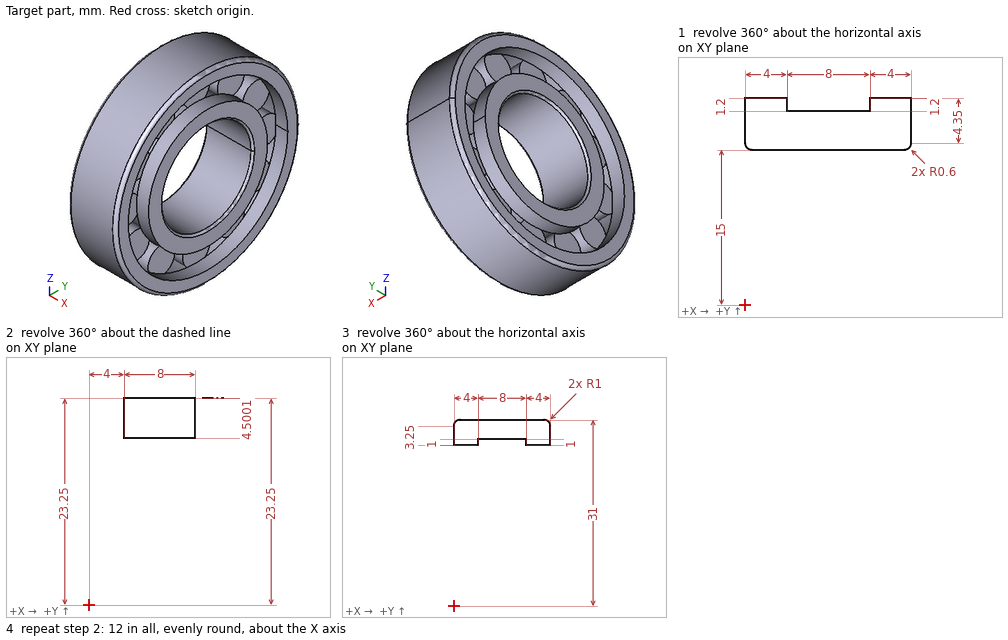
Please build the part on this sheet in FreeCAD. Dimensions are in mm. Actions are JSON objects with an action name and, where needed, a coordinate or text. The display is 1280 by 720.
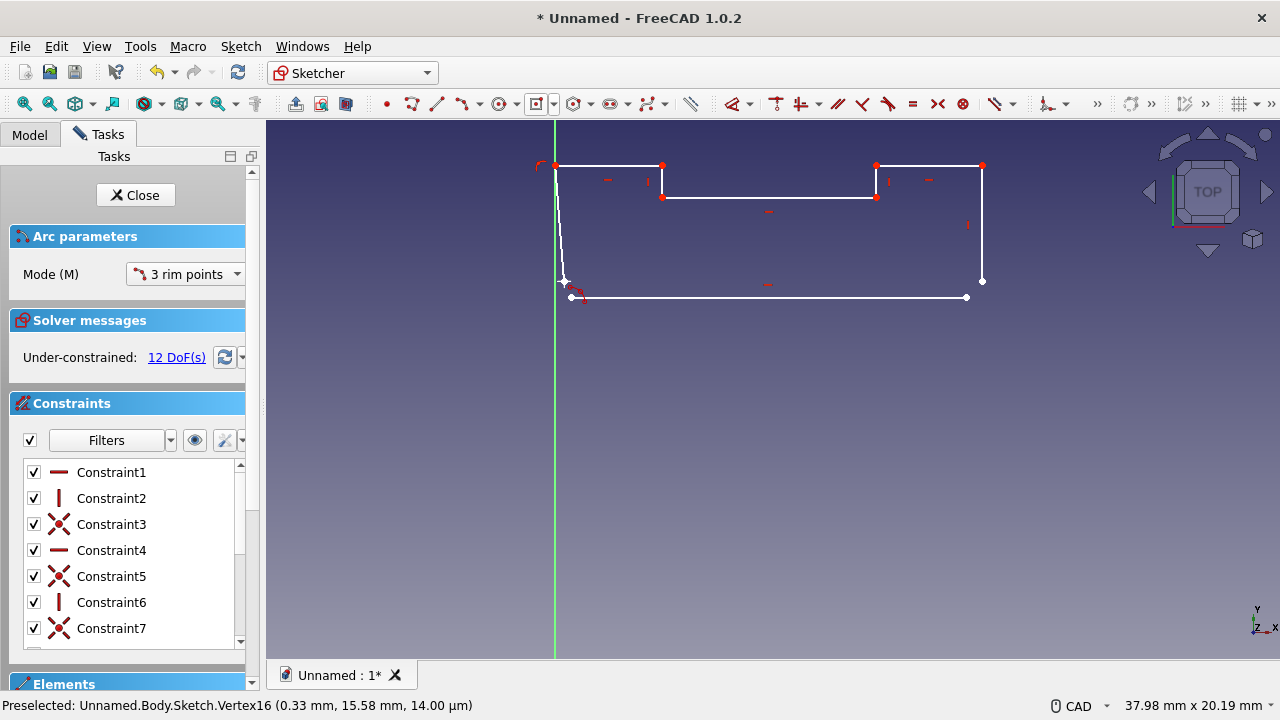
{"action": "left_click", "coordinate": [966, 298]}
{"action": "left_click", "coordinate": [982, 282]}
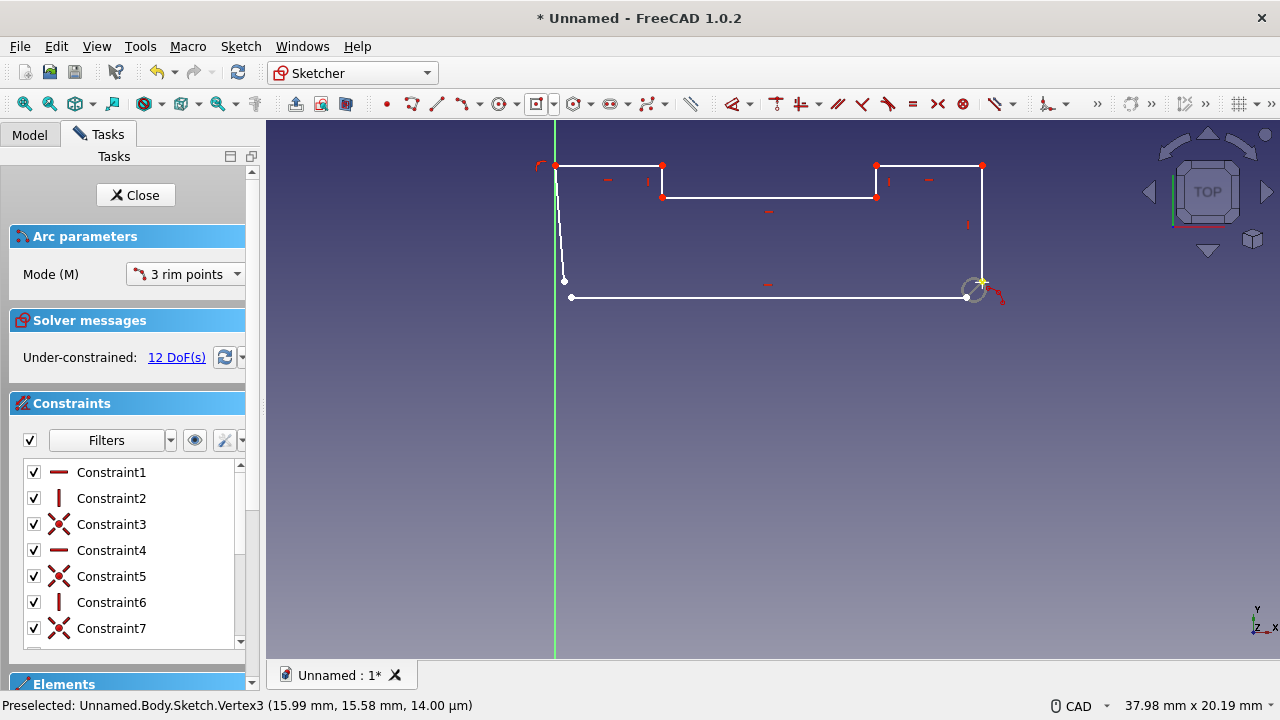
{"action": "scroll", "coordinate": [978, 293], "scroll_direction": "up", "scroll_amount": 7}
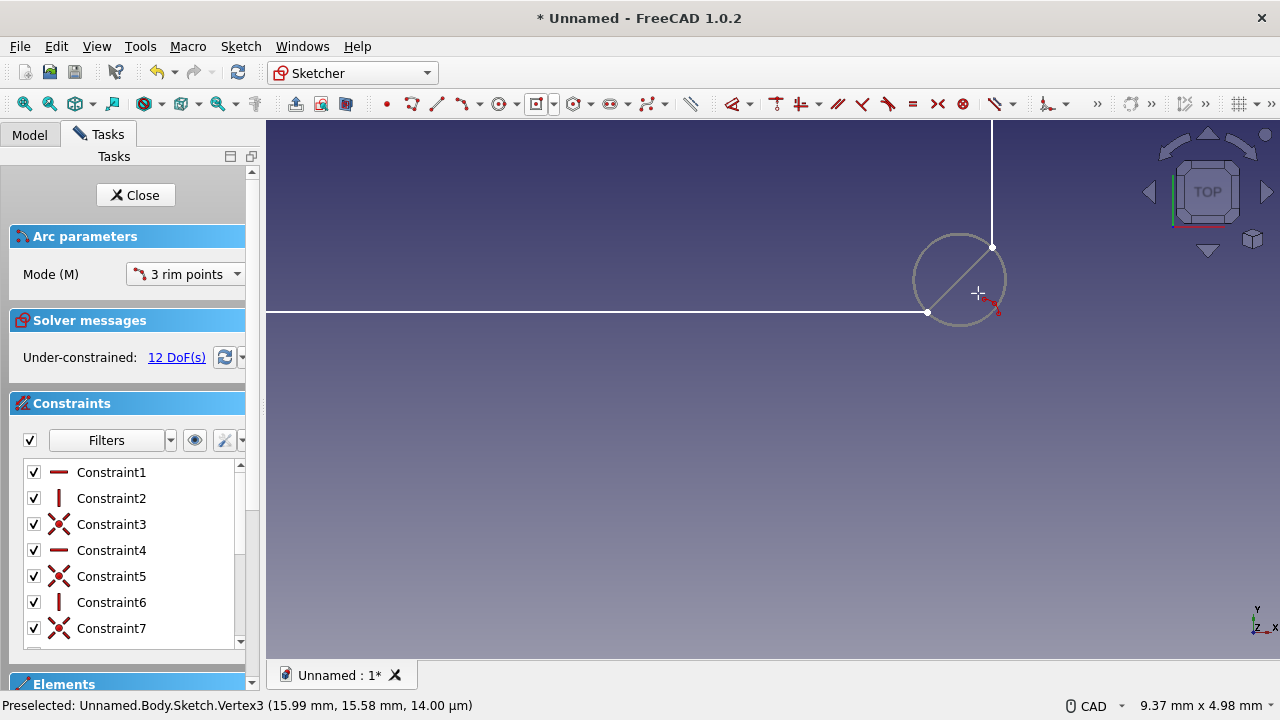
{"action": "left_click", "coordinate": [974, 291]}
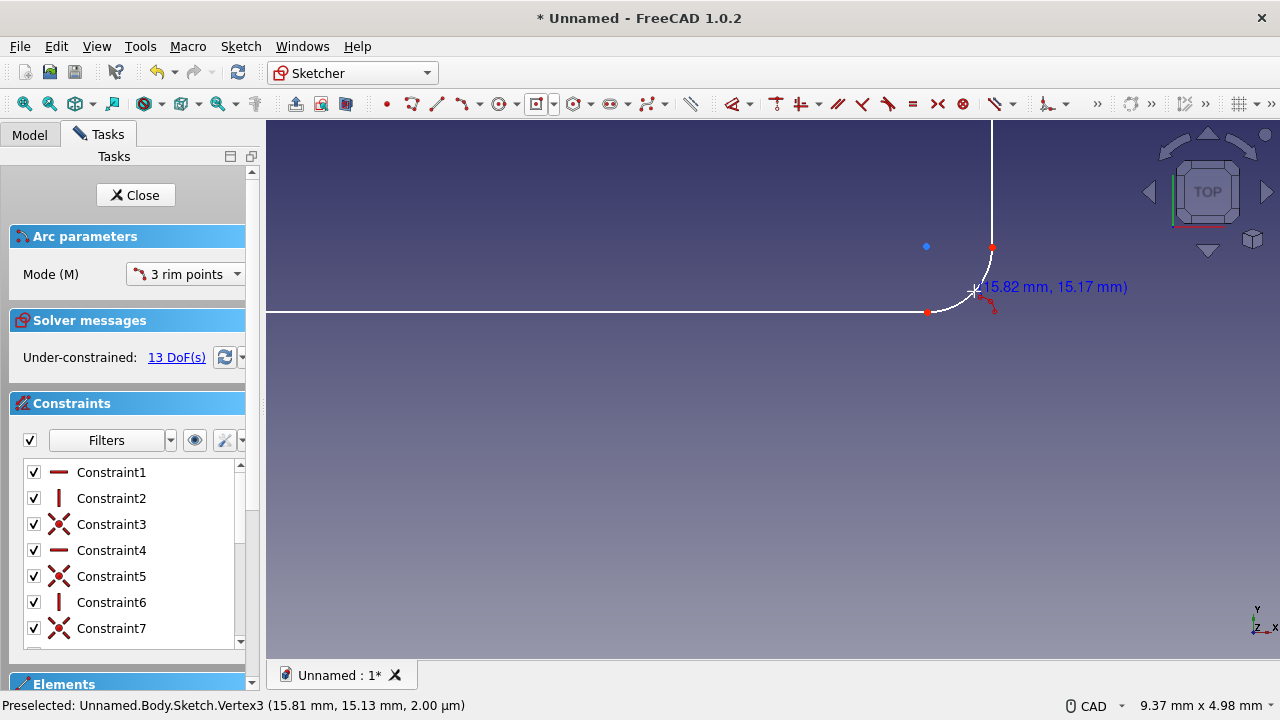
{"action": "scroll", "coordinate": [819, 298], "scroll_direction": "down", "scroll_amount": 9}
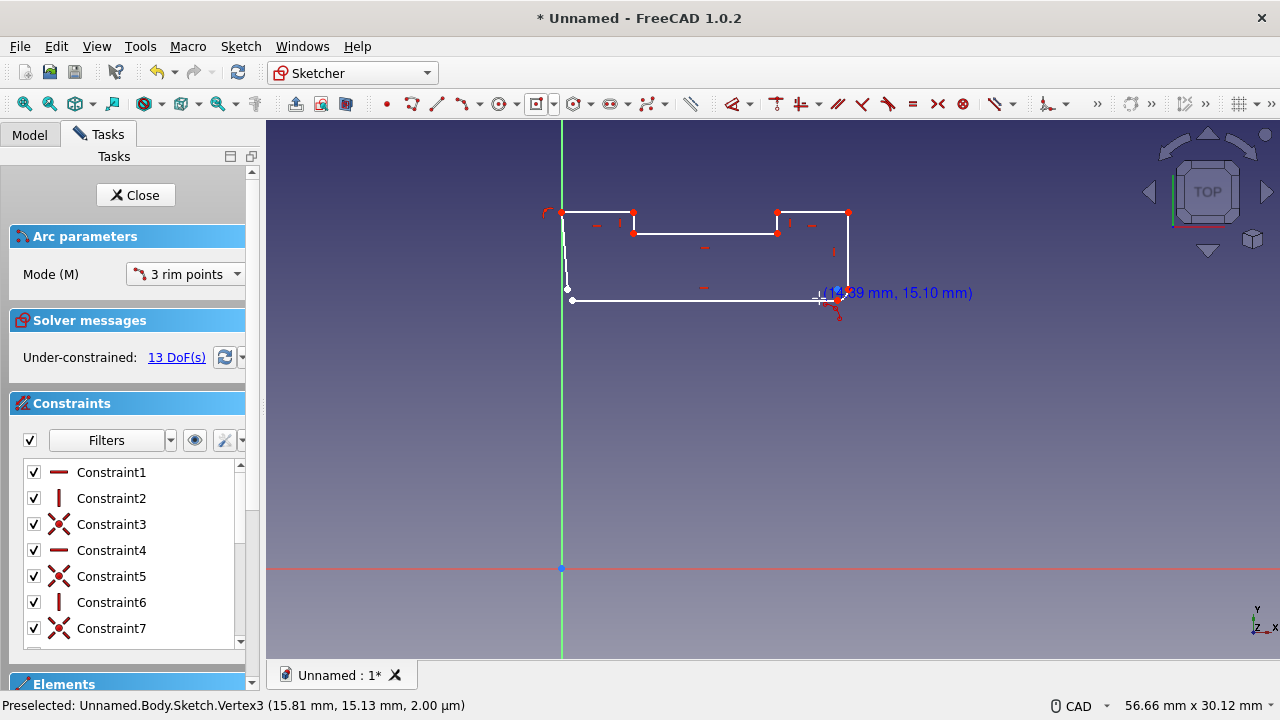
{"action": "left_click", "coordinate": [568, 290]}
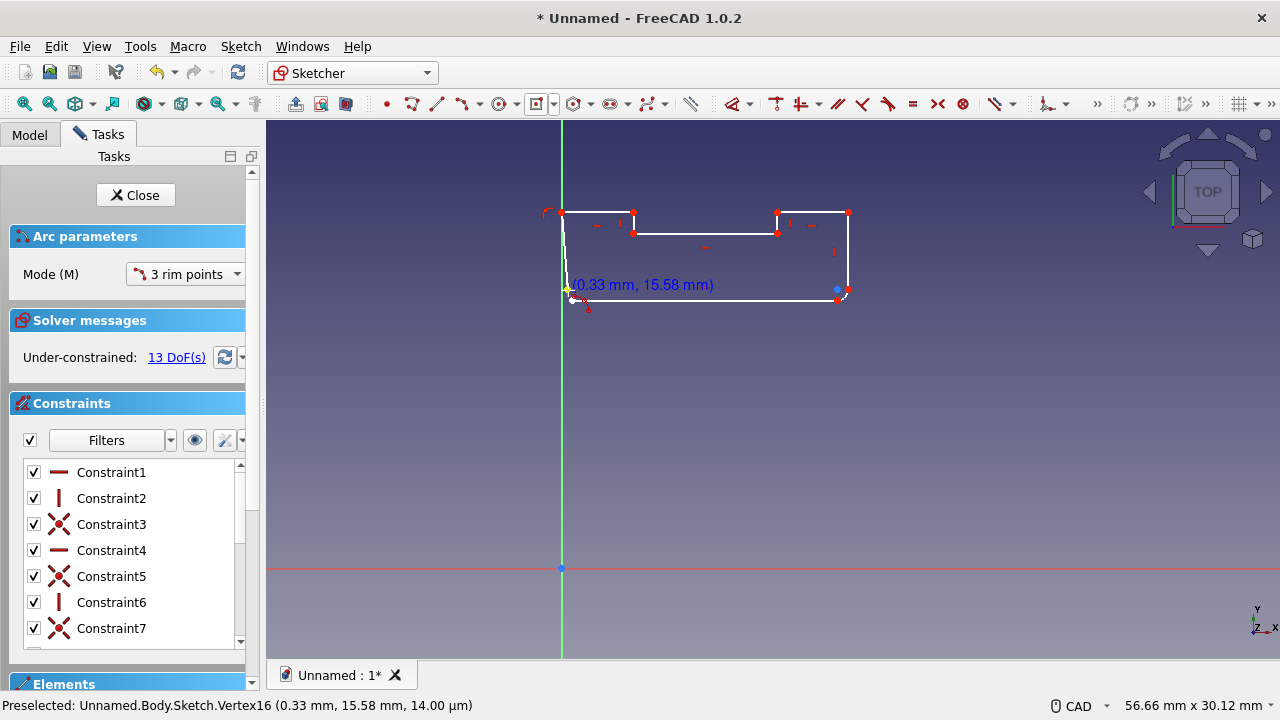
{"action": "scroll", "coordinate": [573, 300], "scroll_direction": "up", "scroll_amount": 2}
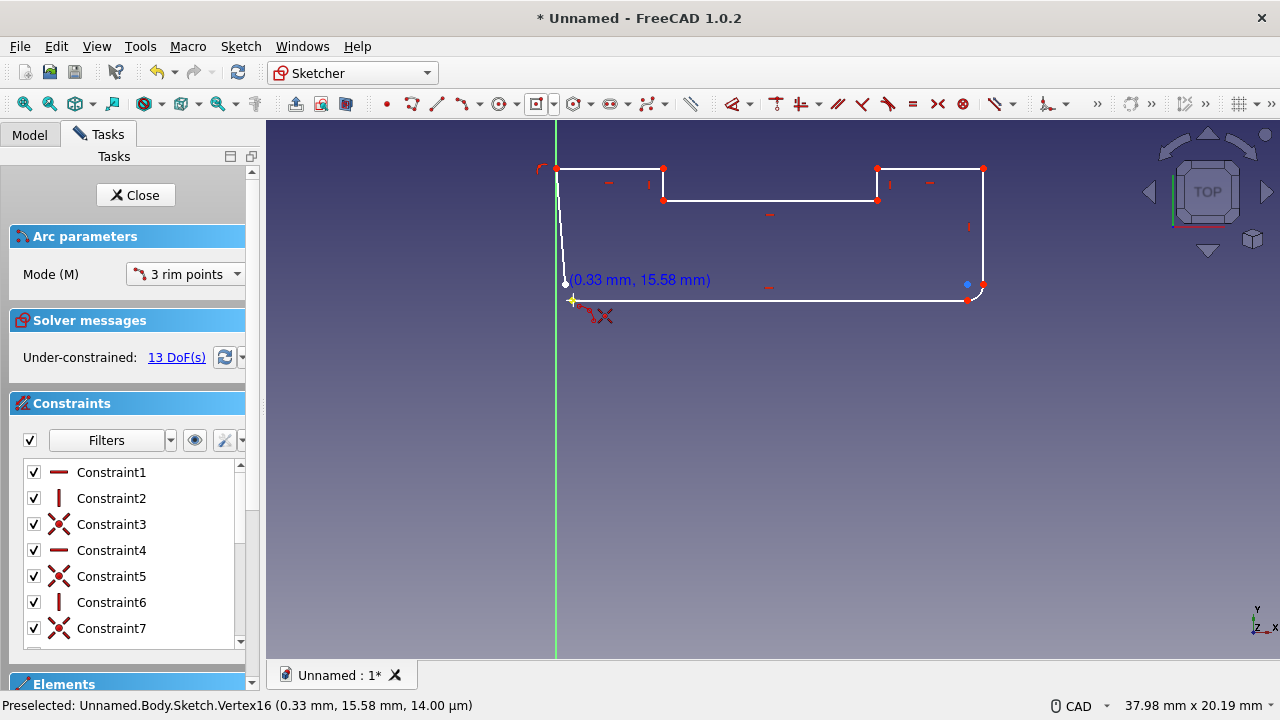
{"action": "left_click", "coordinate": [572, 301]}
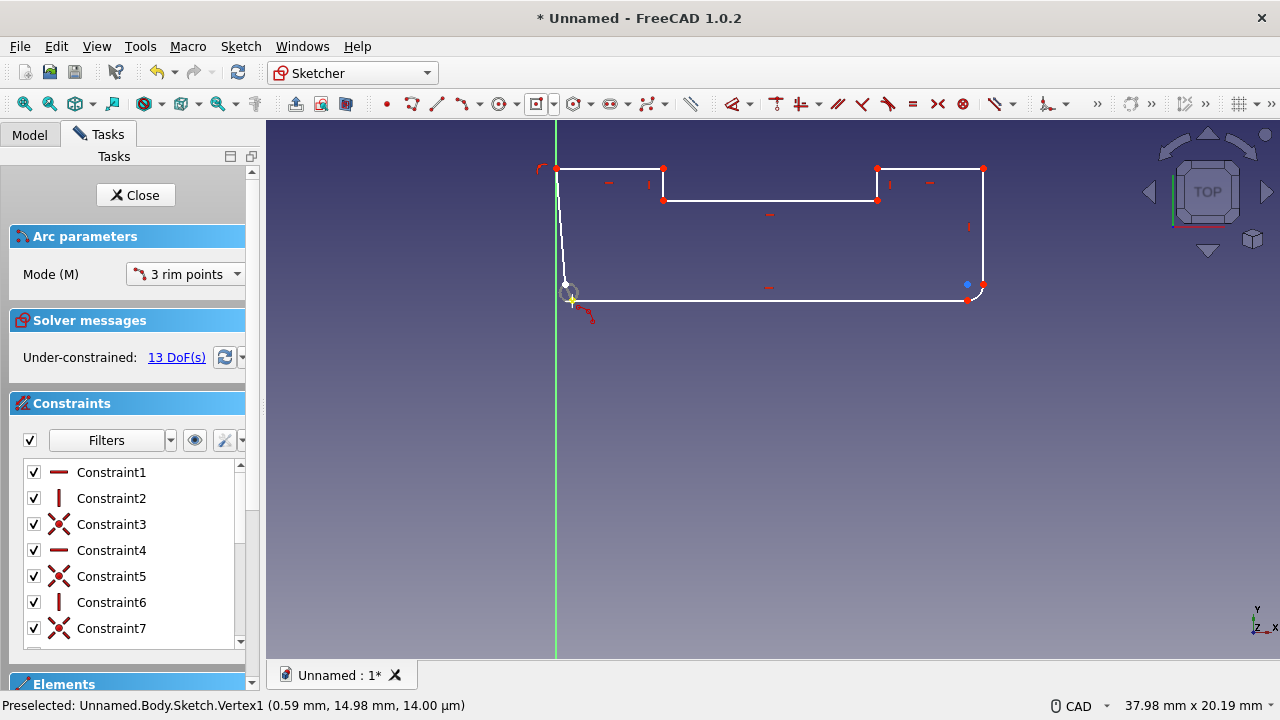
{"action": "scroll", "coordinate": [561, 296], "scroll_direction": "up", "scroll_amount": 7}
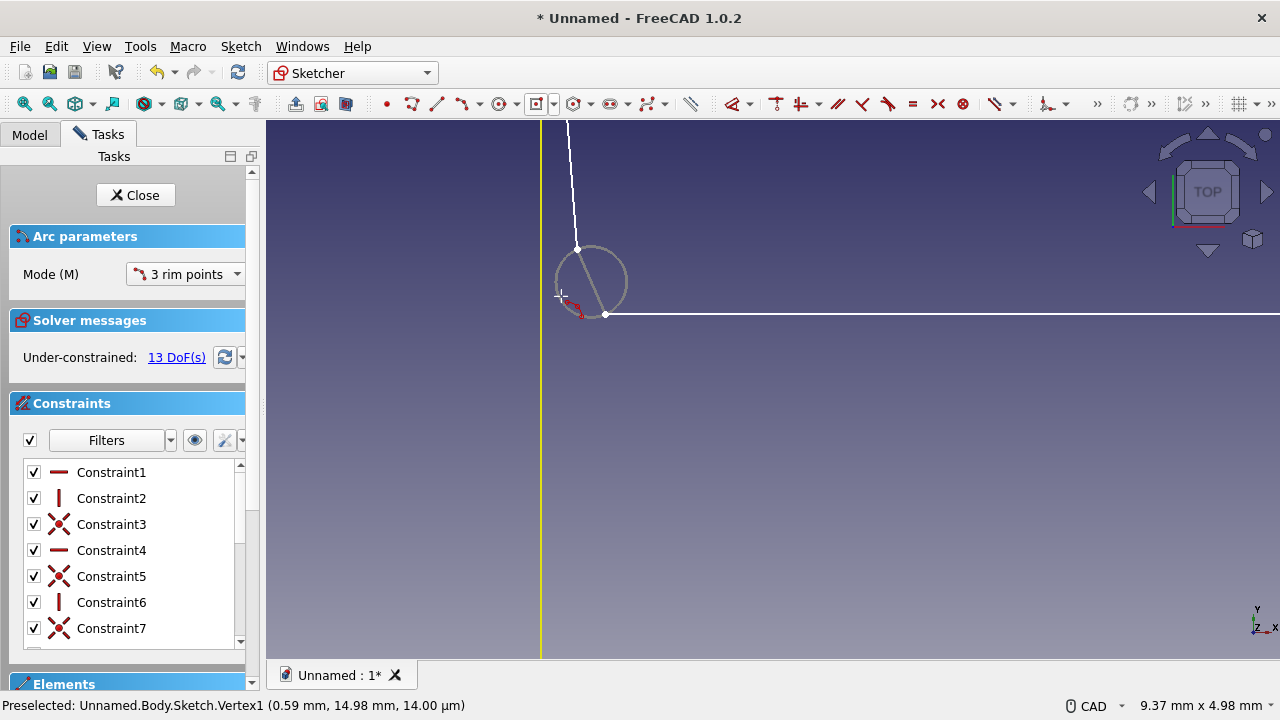
{"action": "left_click", "coordinate": [560, 293]}
{"action": "key", "text": "Escape"}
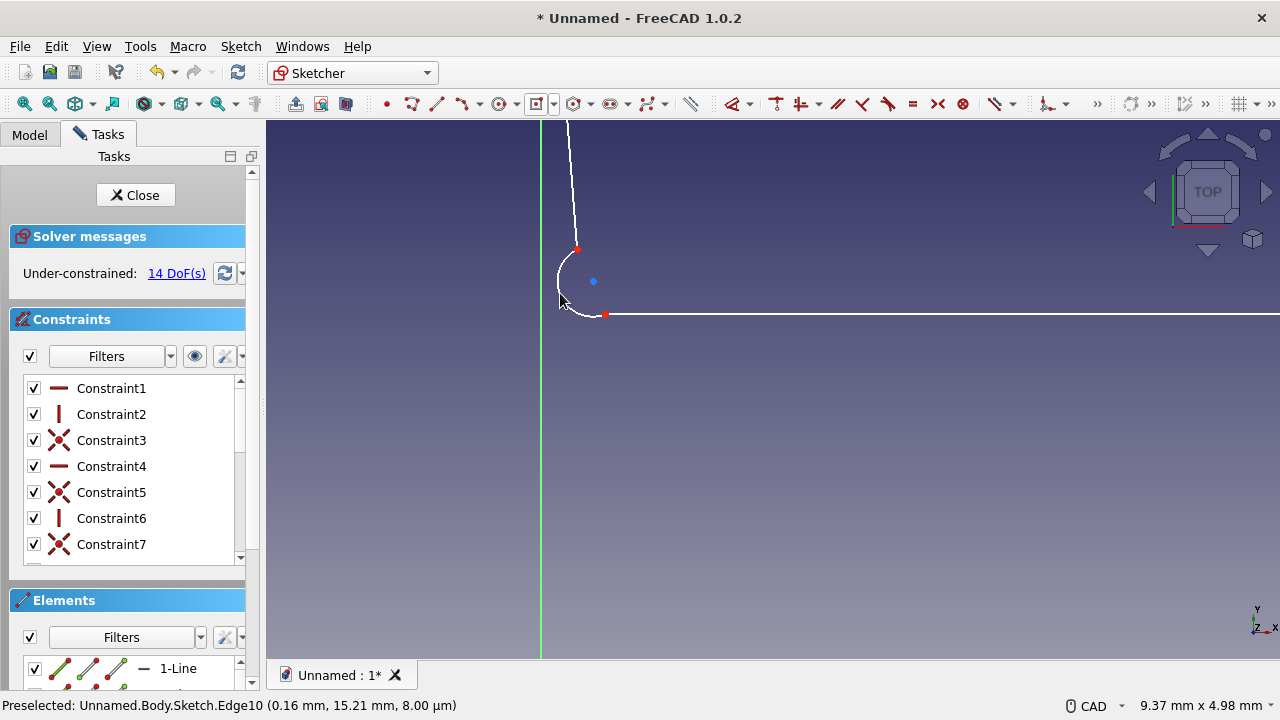
{"action": "scroll", "coordinate": [565, 297], "scroll_direction": "down", "scroll_amount": 9}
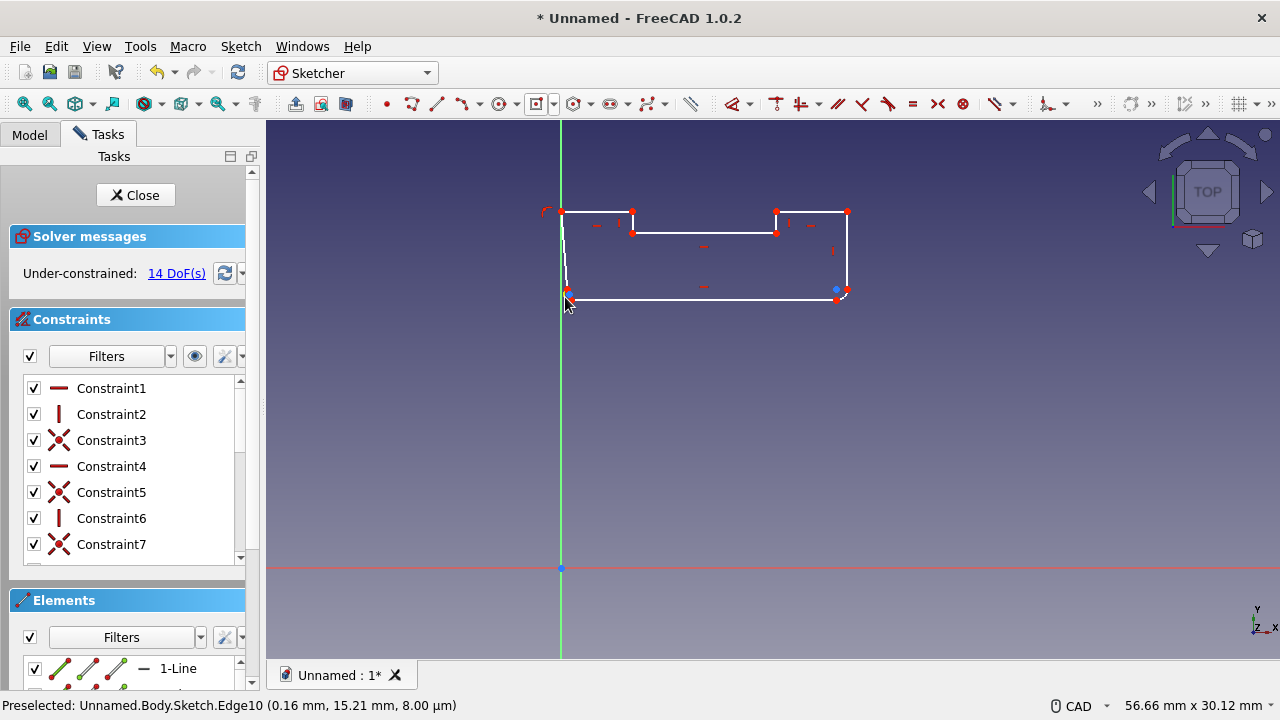
{"action": "left_click", "coordinate": [651, 300]}